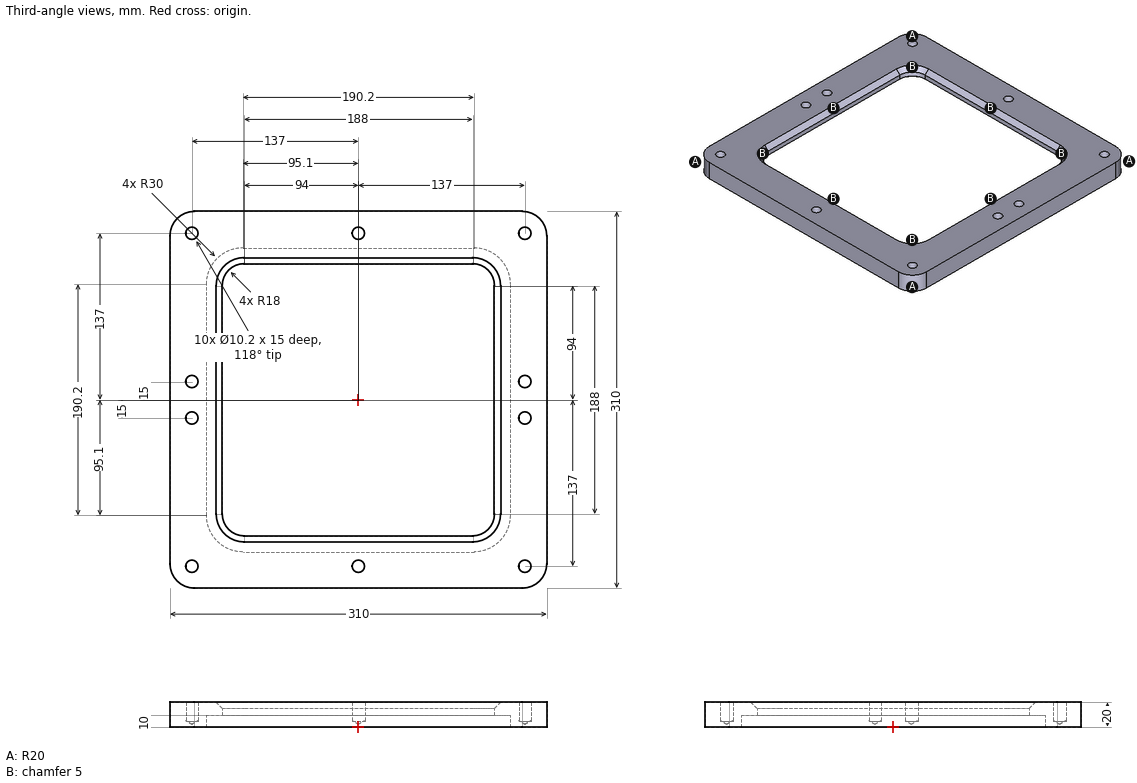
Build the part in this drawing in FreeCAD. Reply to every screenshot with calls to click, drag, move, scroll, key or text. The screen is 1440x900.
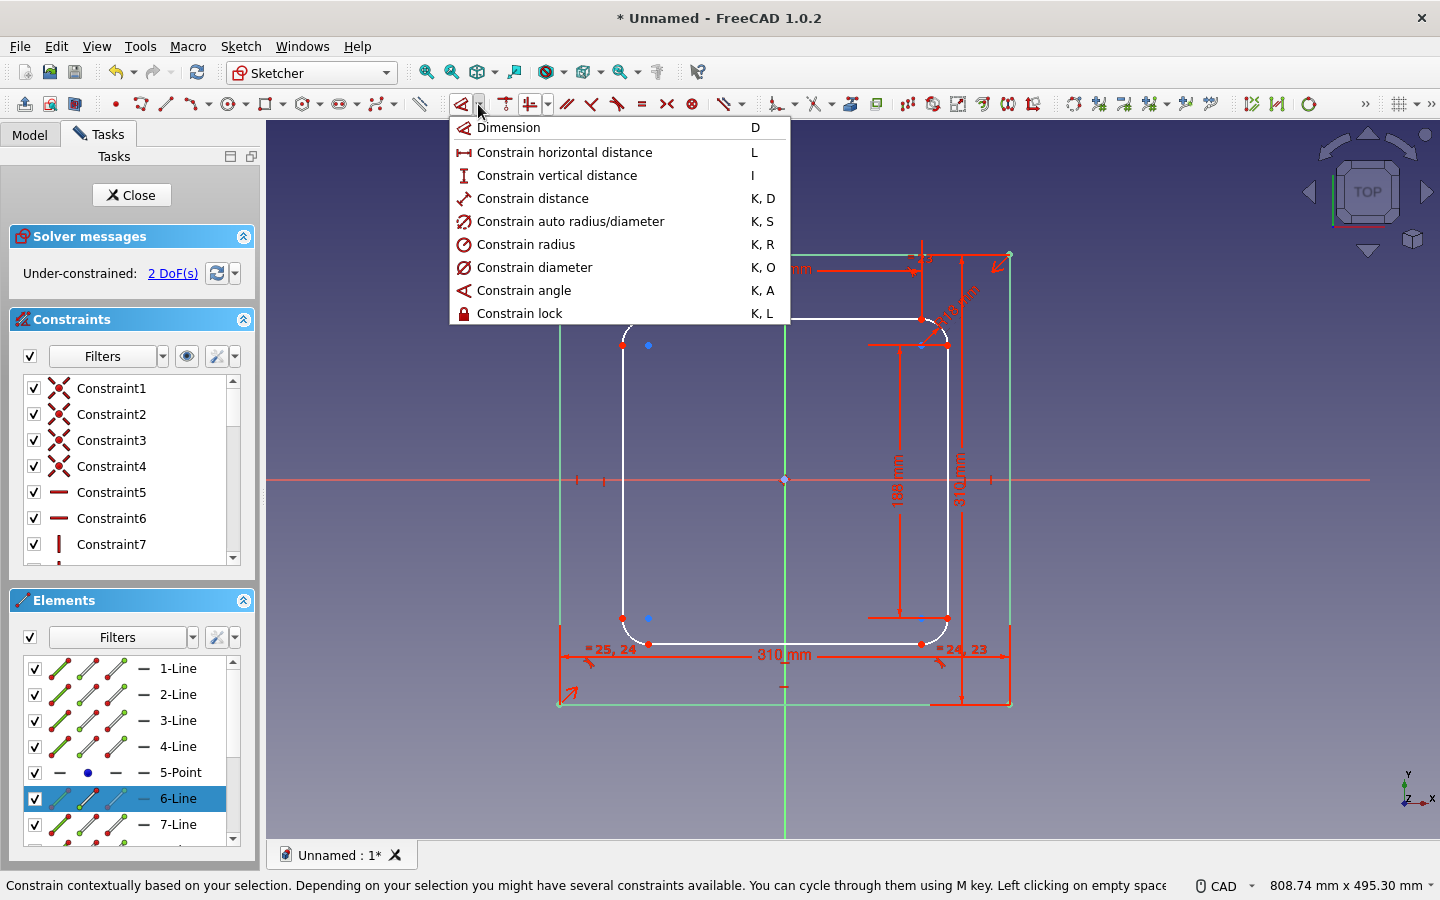
click(620, 152)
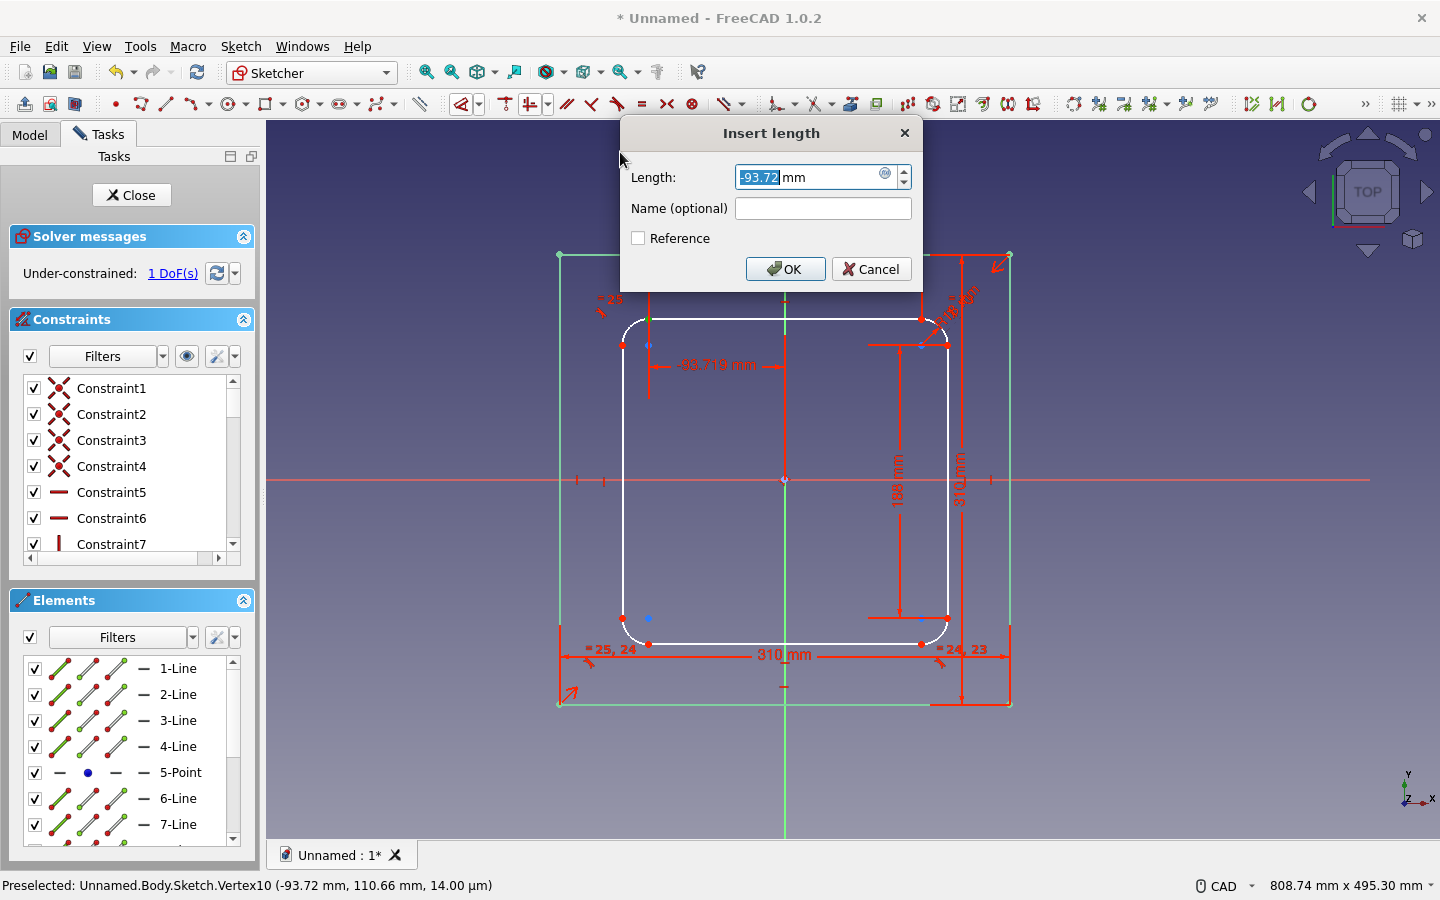
text(-94)
key(Return)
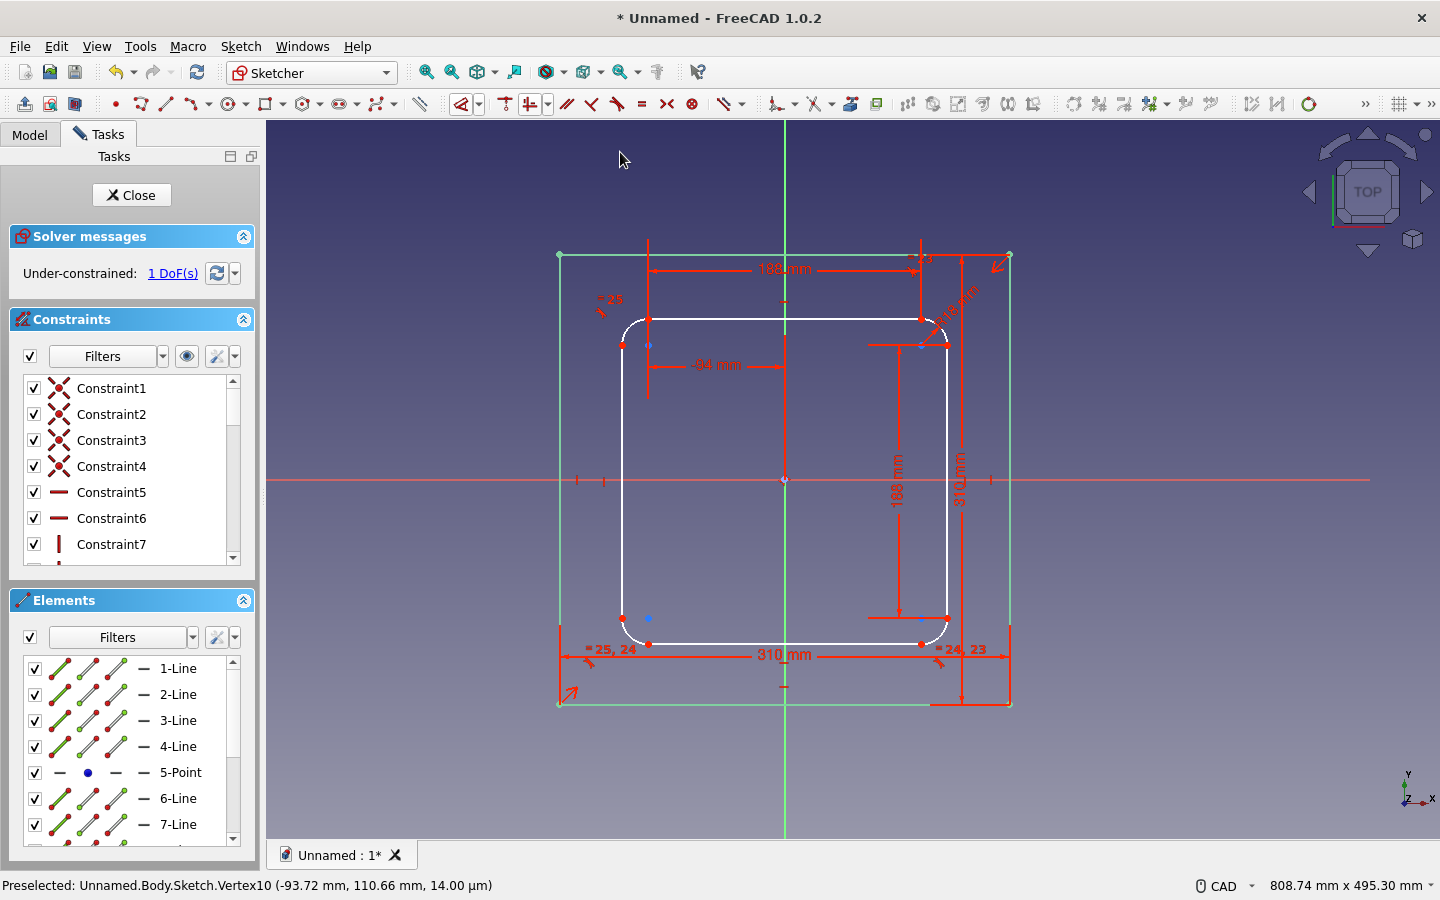
click(947, 345)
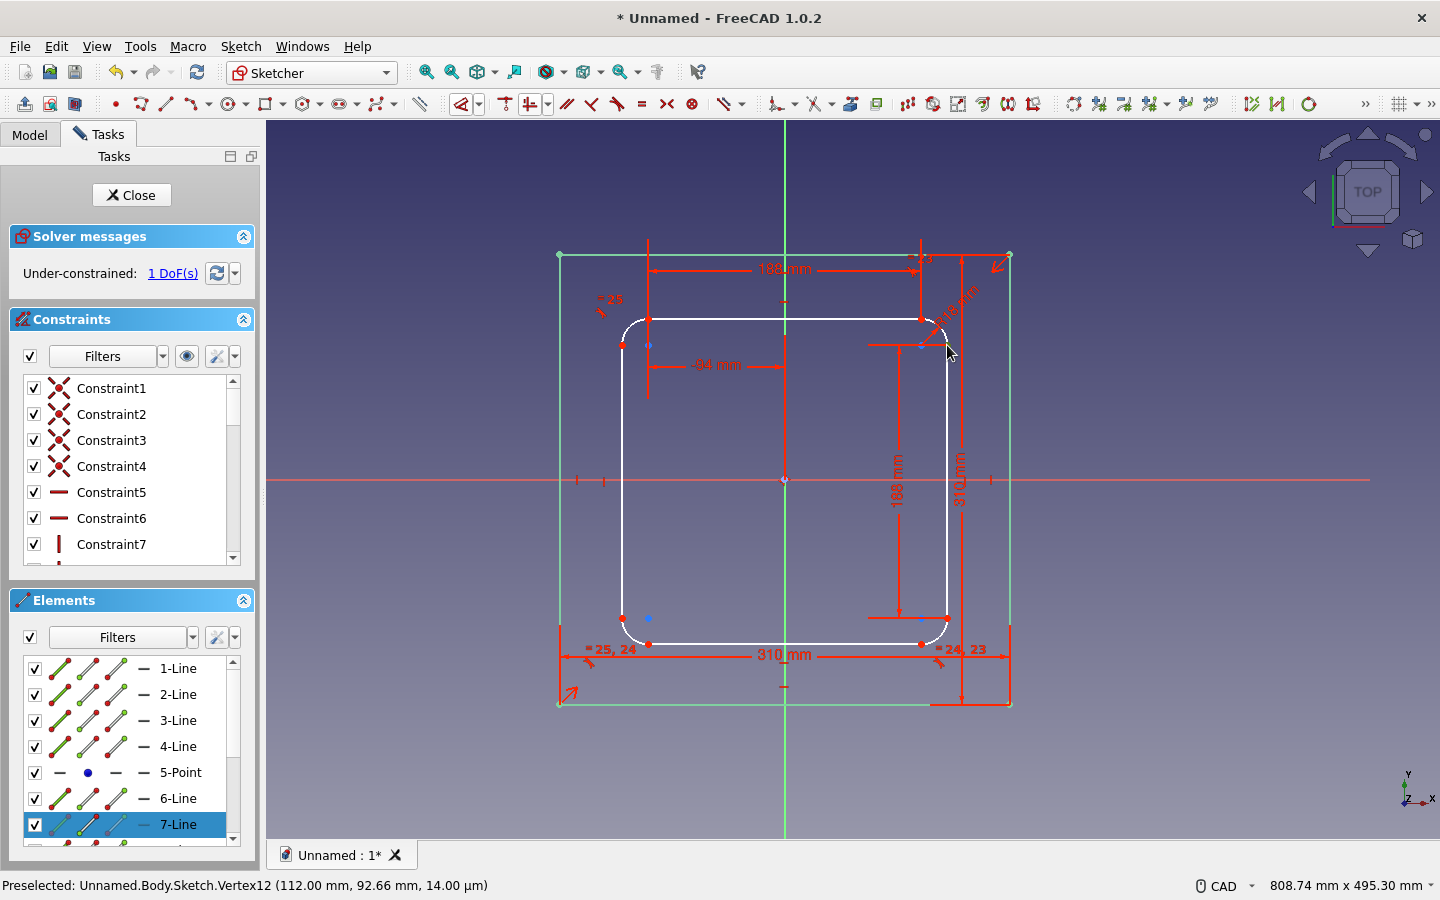
click(478, 104)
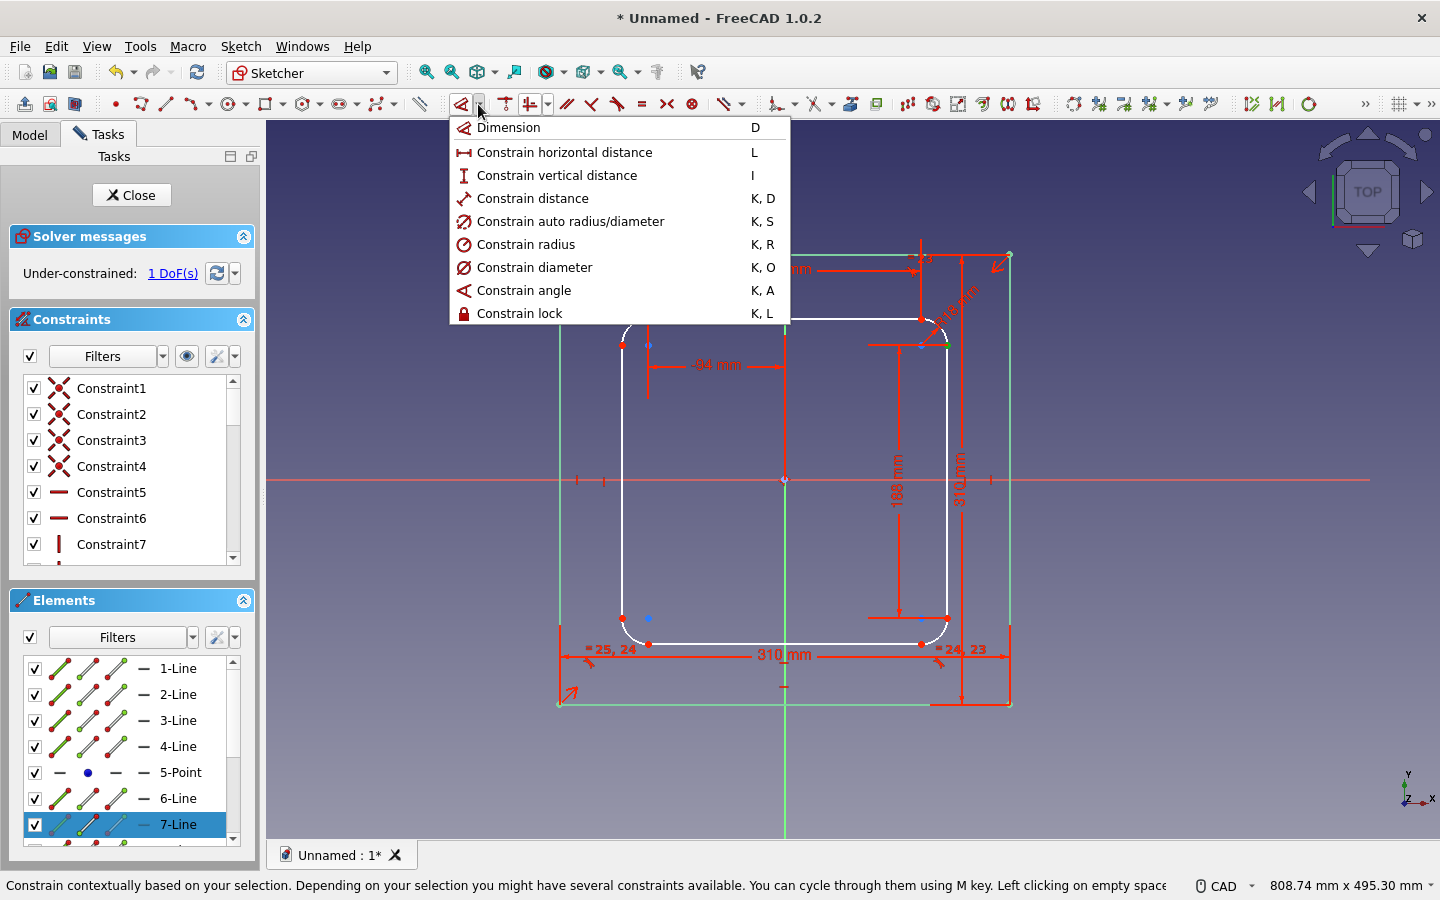
click(620, 176)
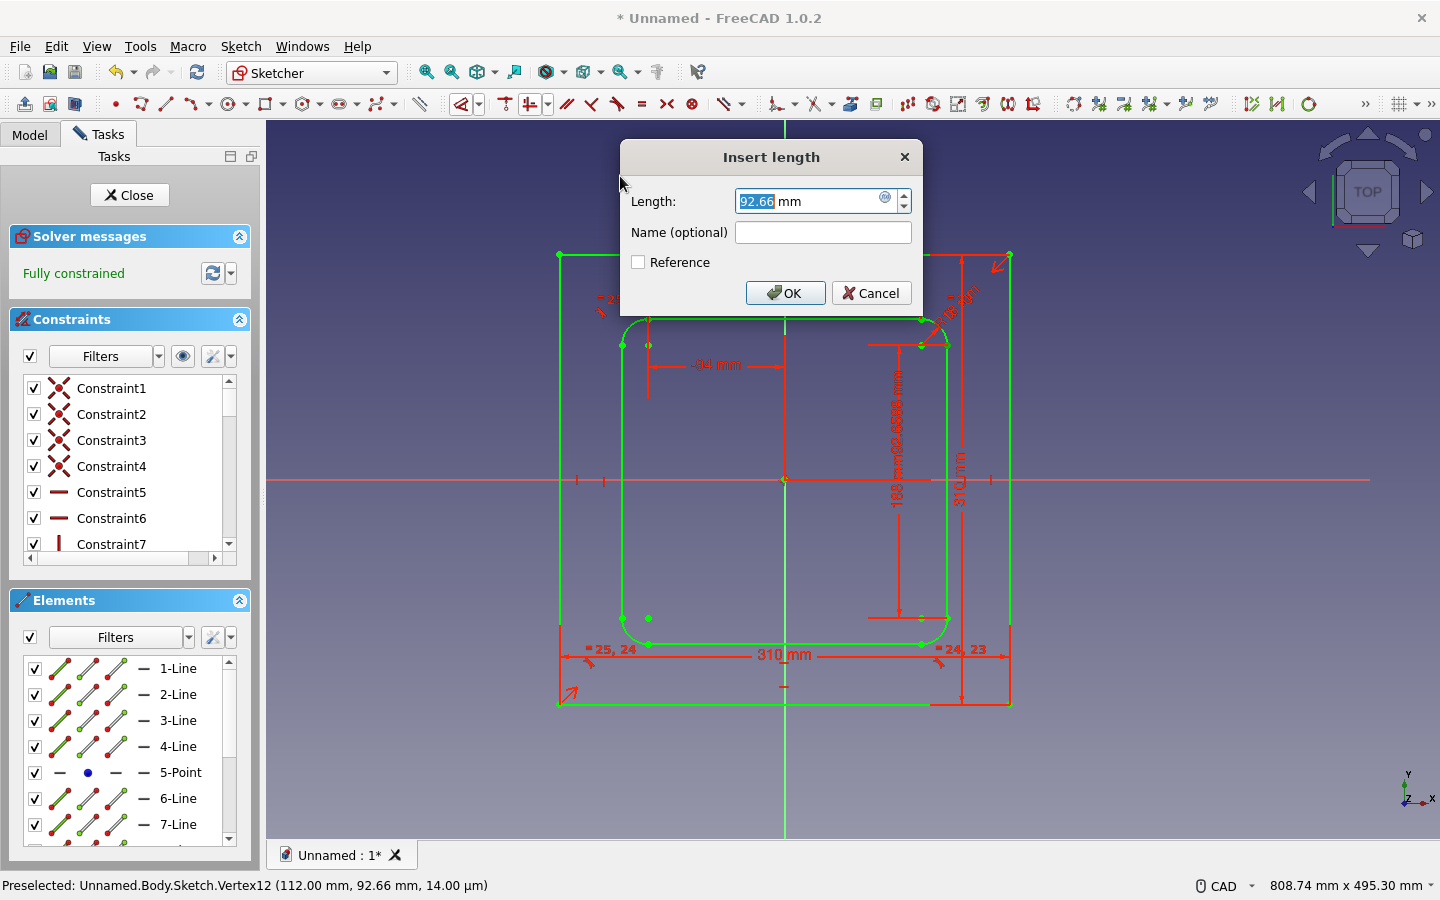
text(94)
key(Return)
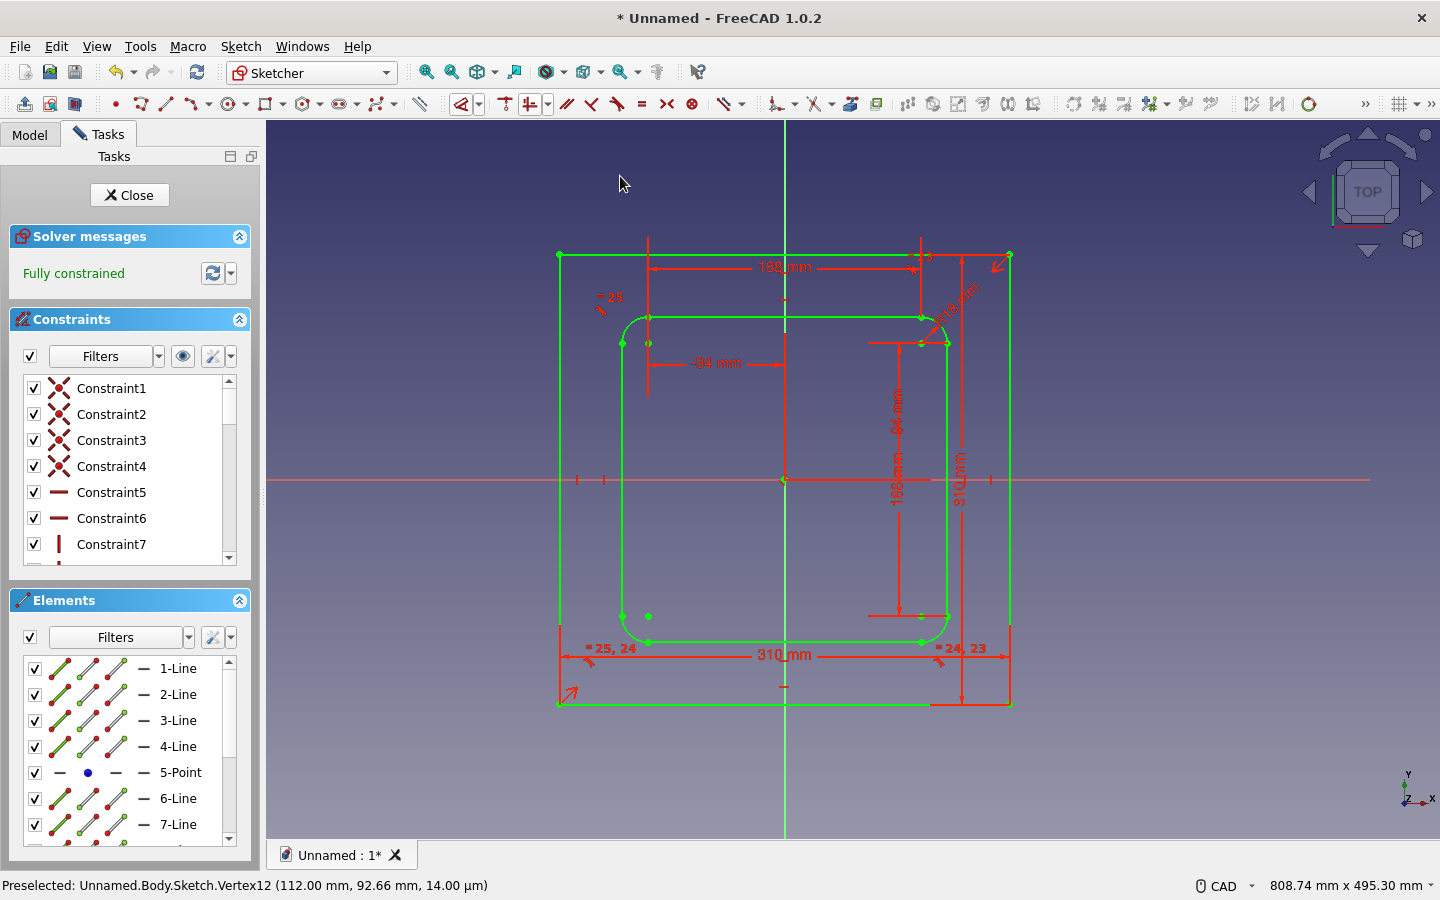
click(130, 195)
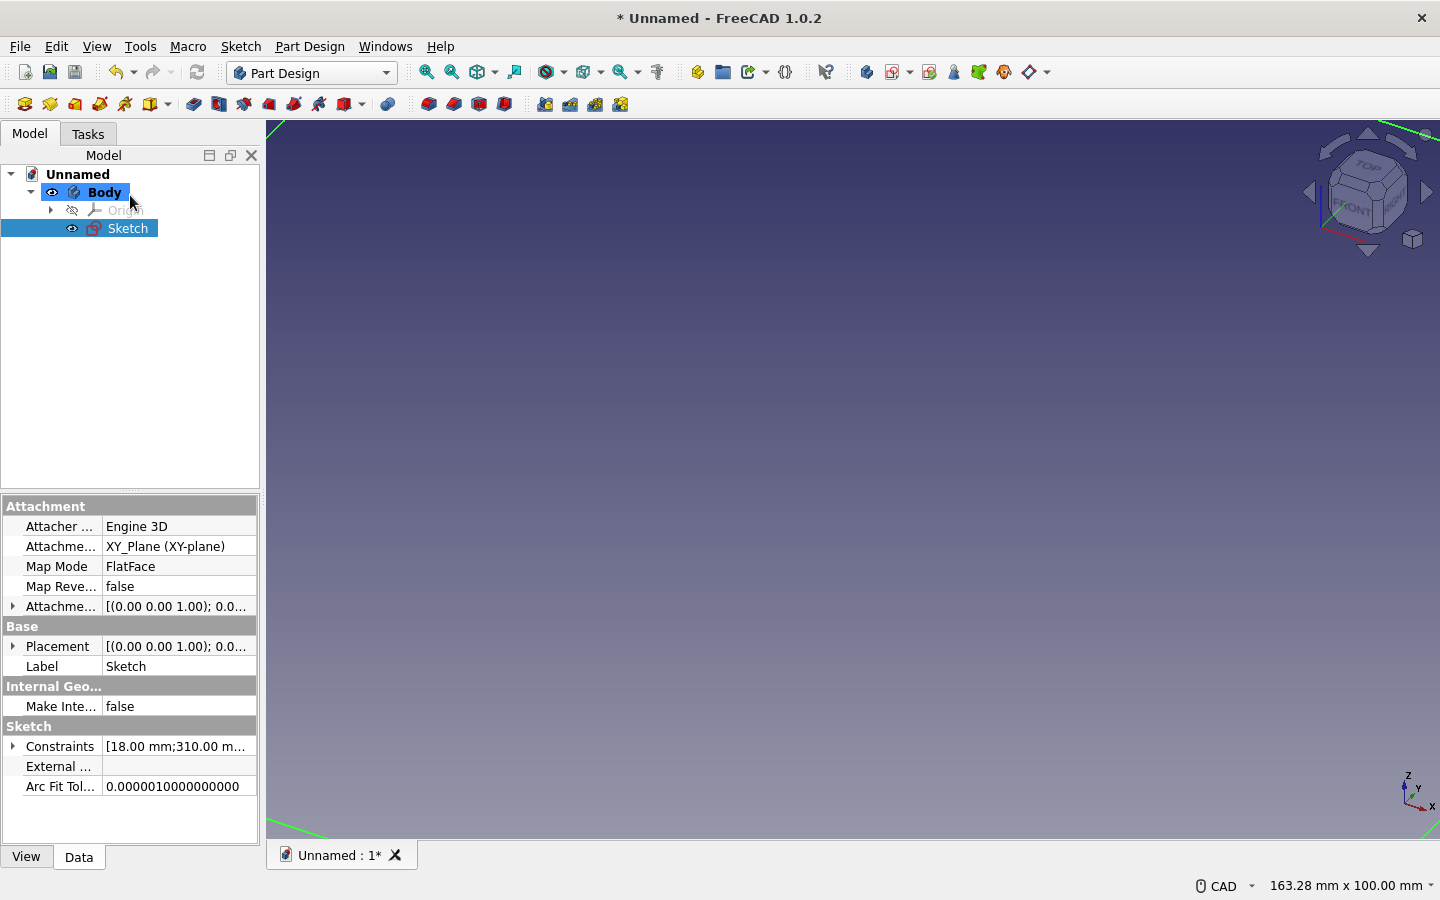
click(25, 104)